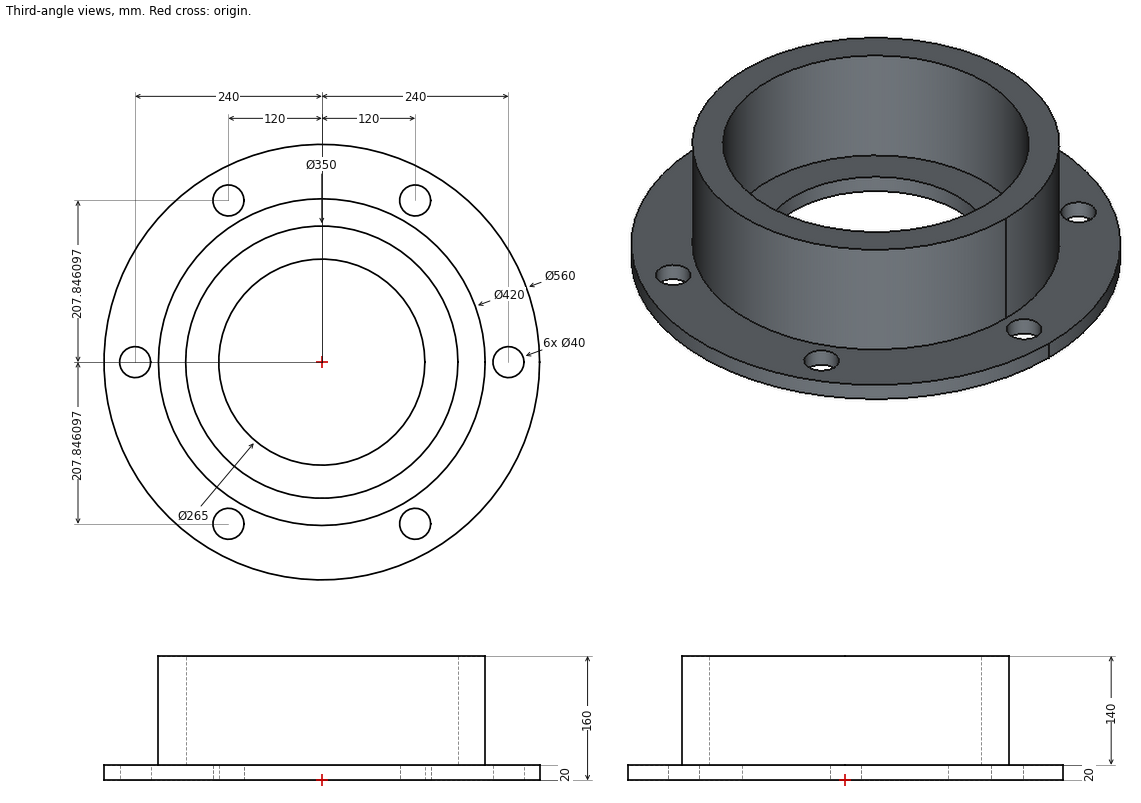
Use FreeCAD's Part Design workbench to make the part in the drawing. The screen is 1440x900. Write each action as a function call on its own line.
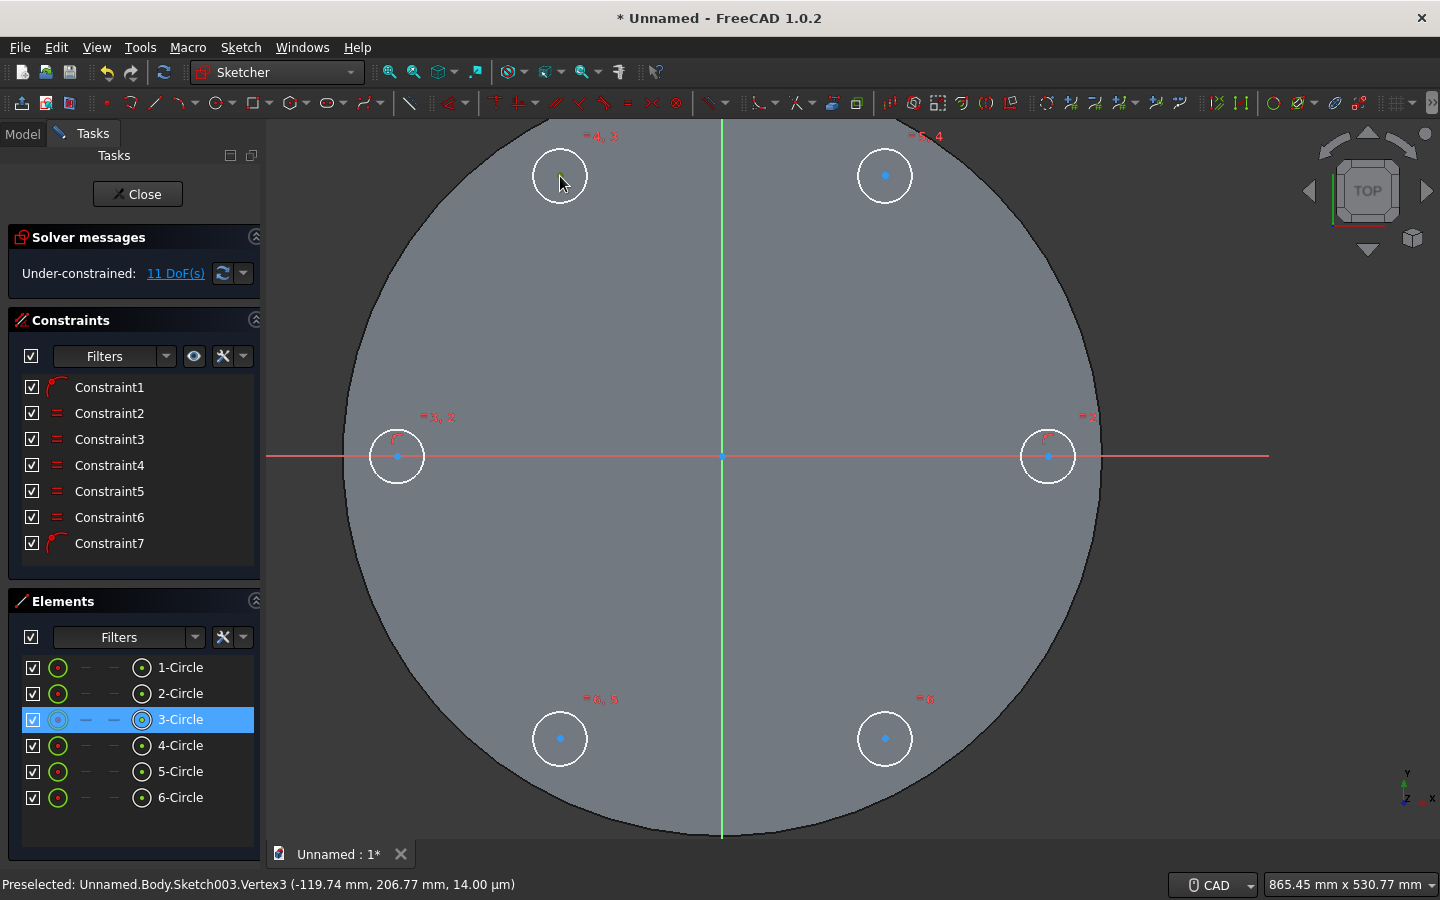
click(885, 176)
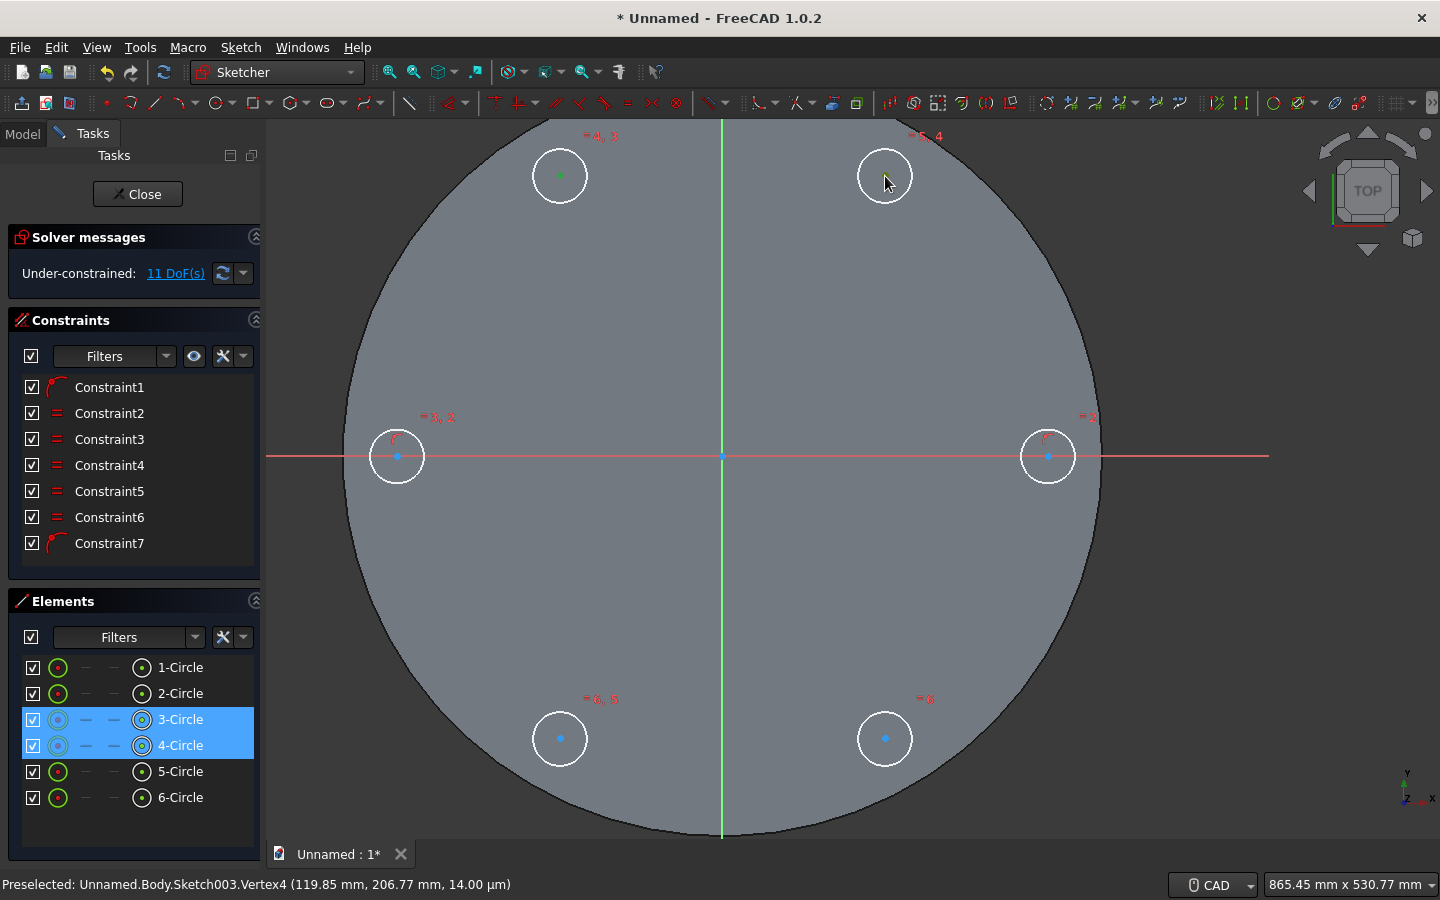
key(h)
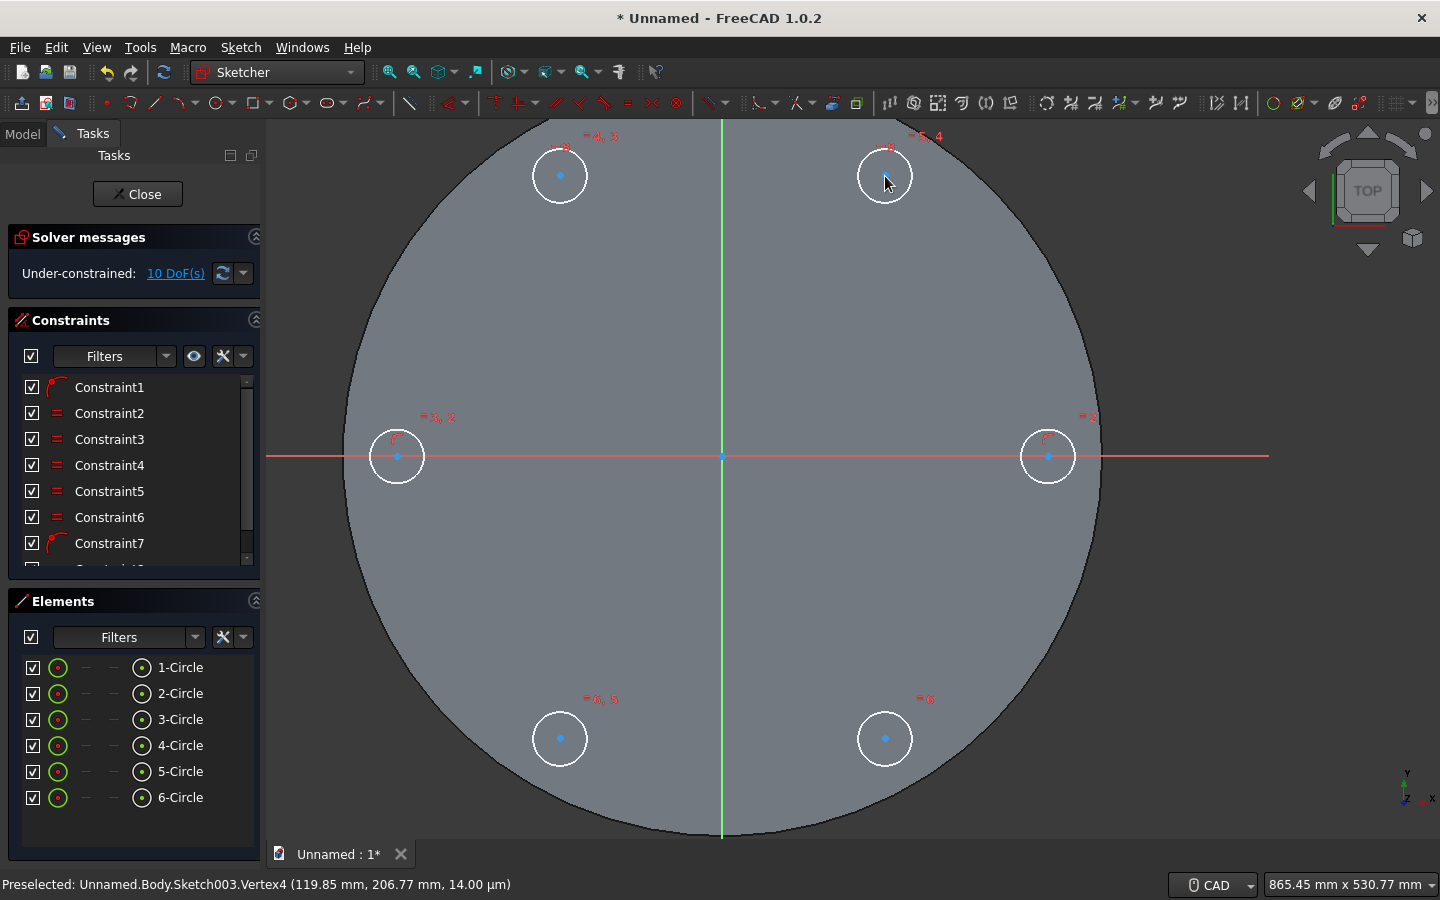
click(560, 176)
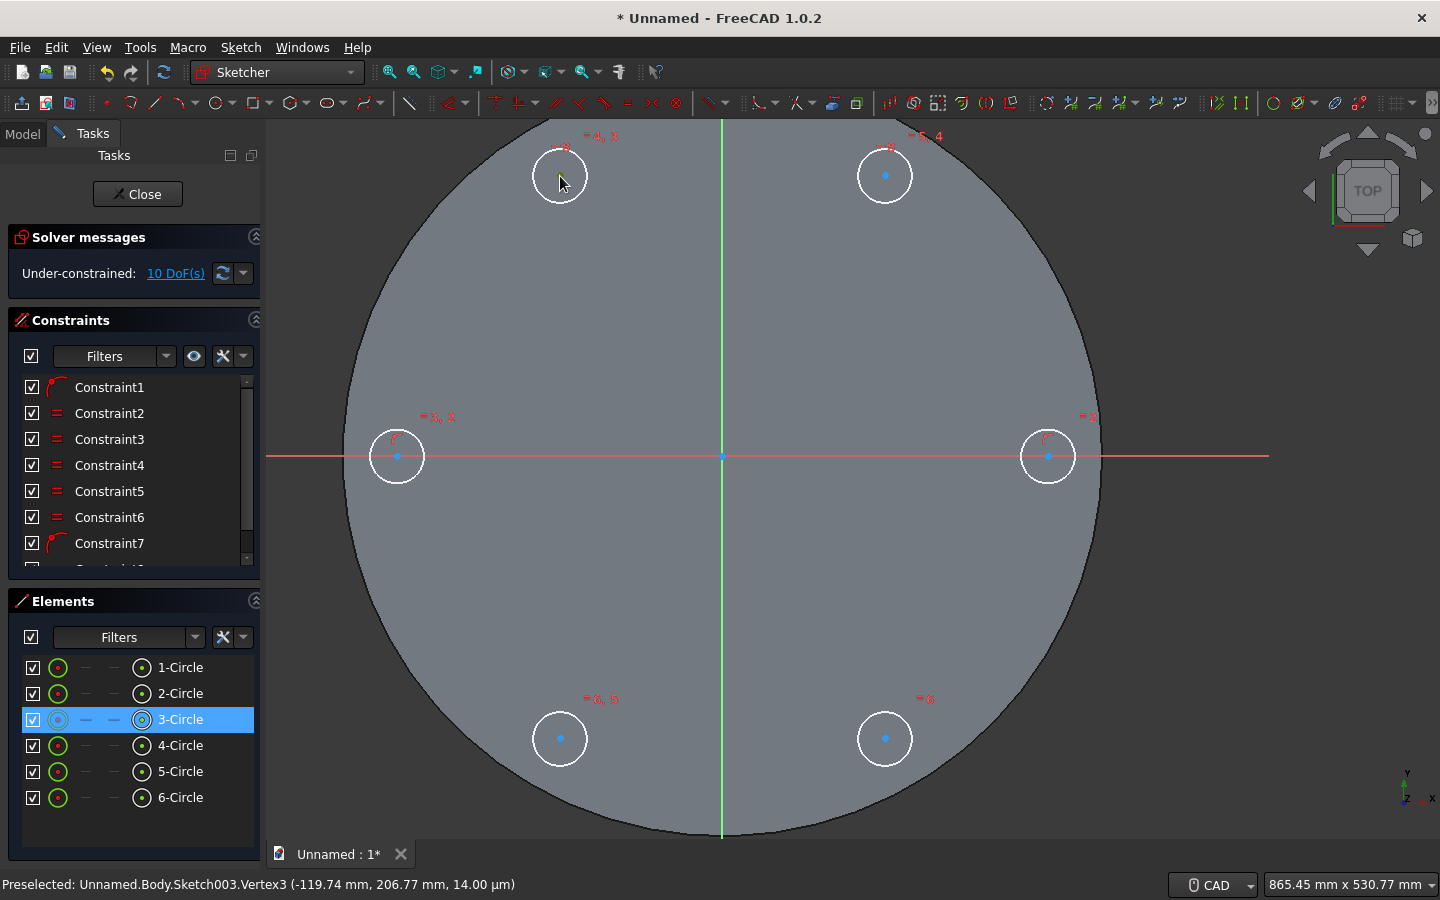
click(560, 739)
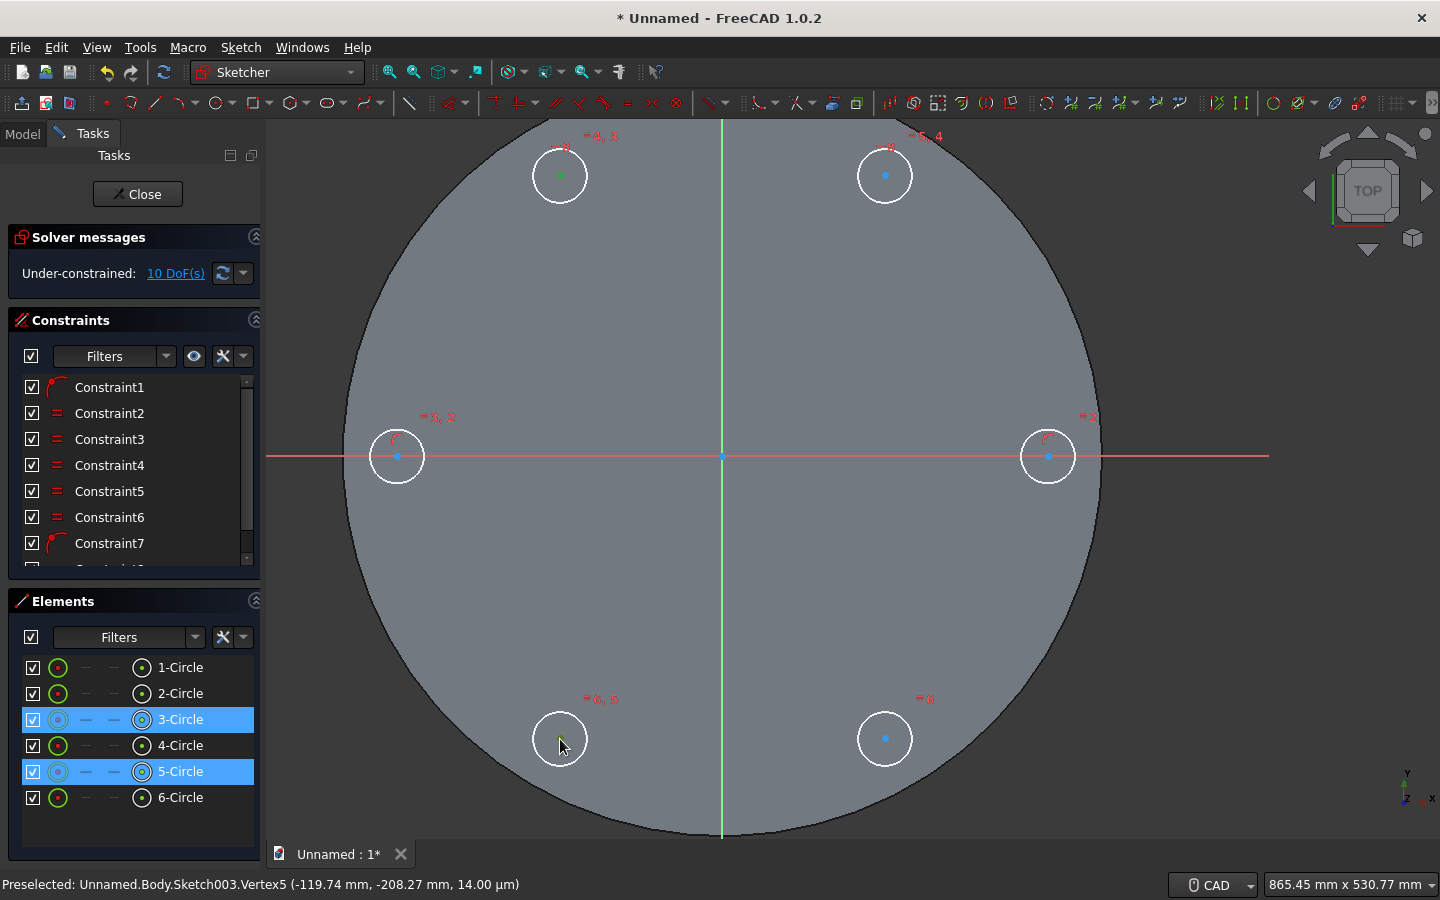
click(538, 104)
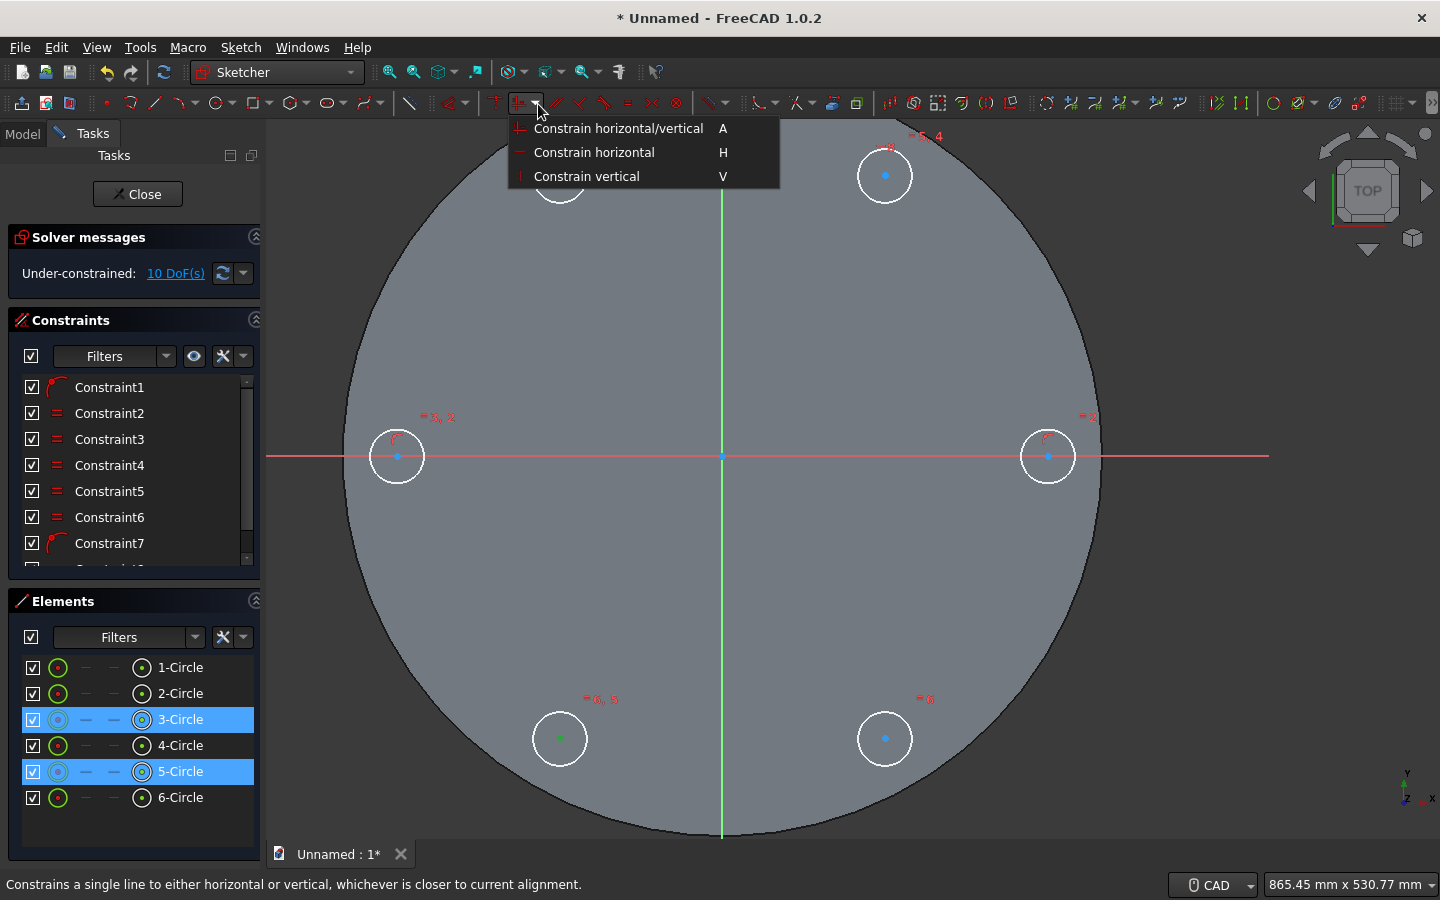
click(644, 176)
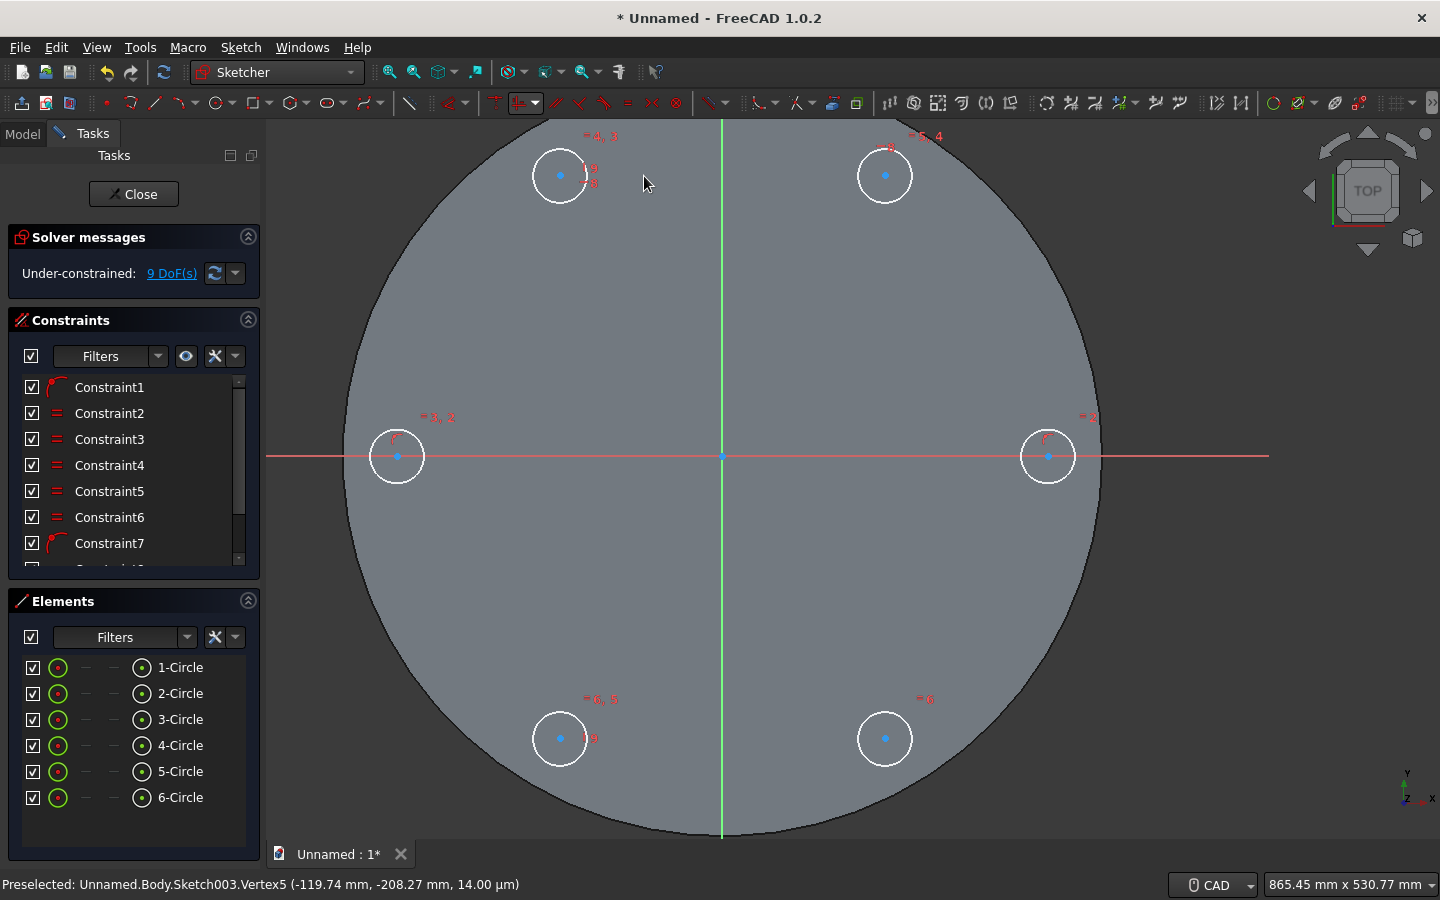
click(885, 176)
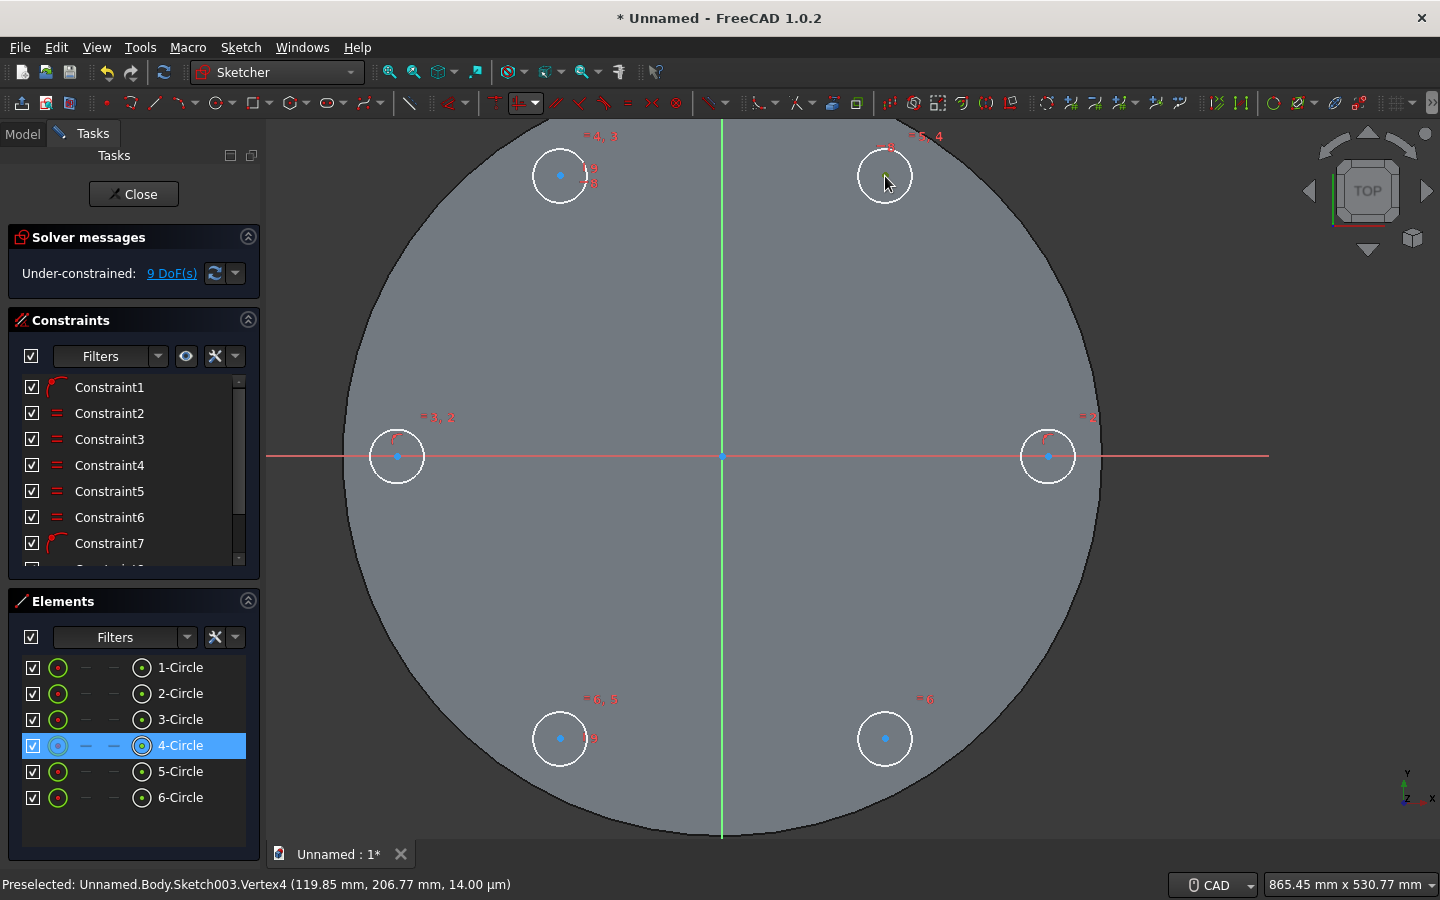
click(885, 739)